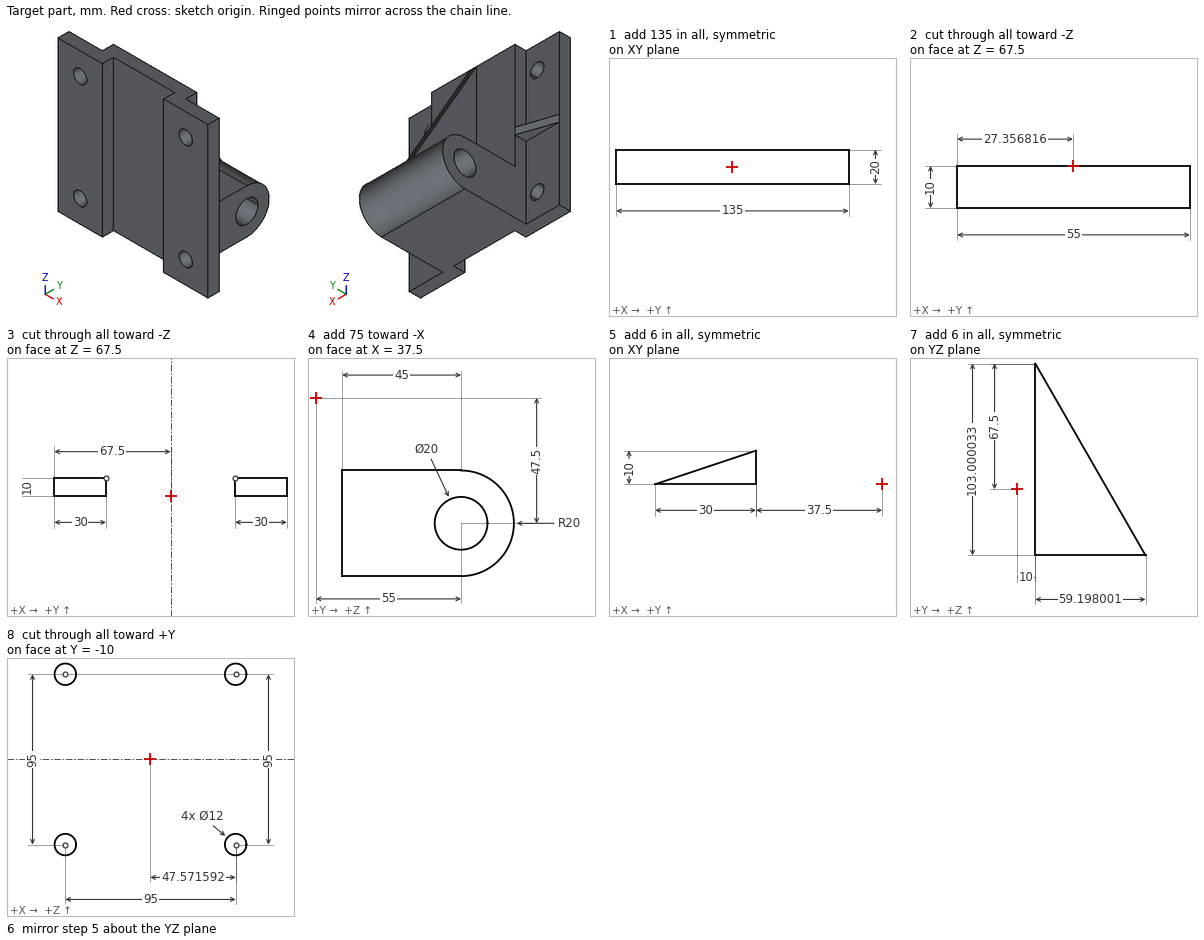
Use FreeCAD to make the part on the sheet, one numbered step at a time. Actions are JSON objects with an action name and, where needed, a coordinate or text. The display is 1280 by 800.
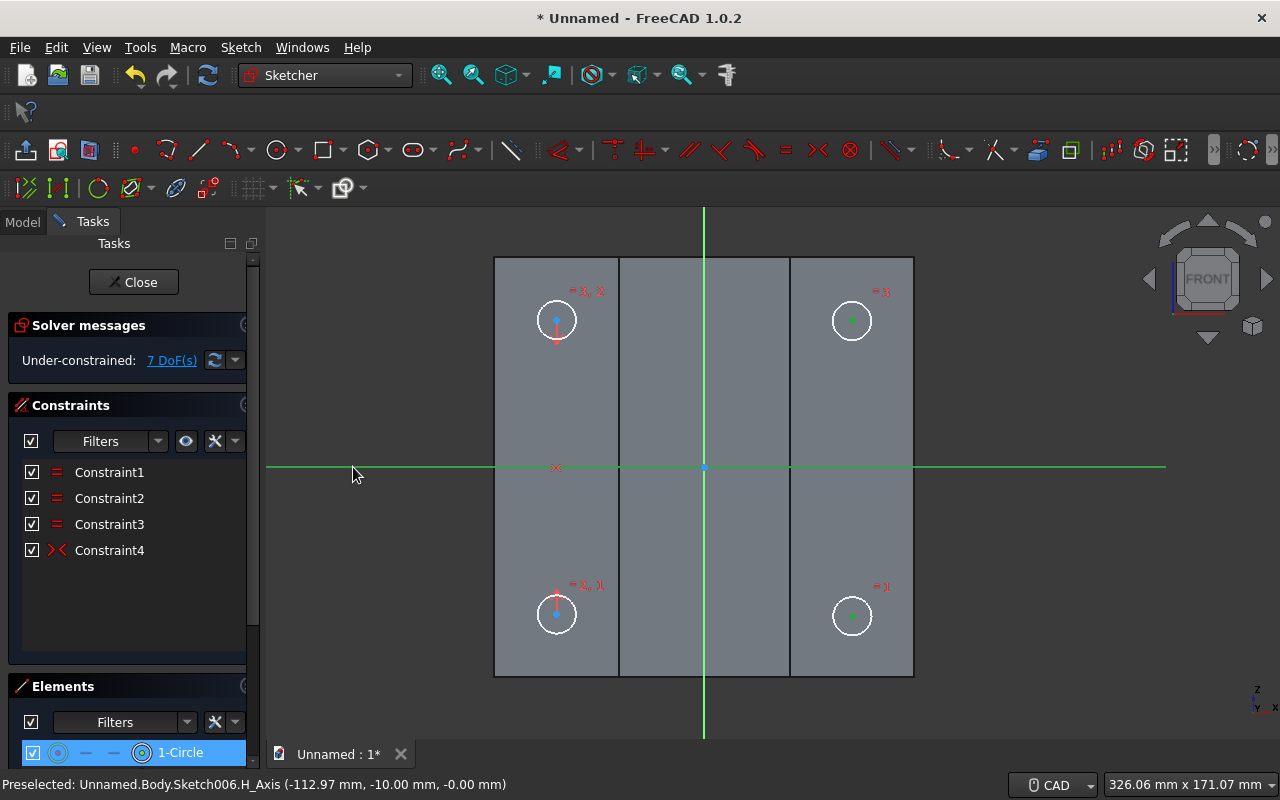
{"action": "left_click", "coordinate": [818, 150]}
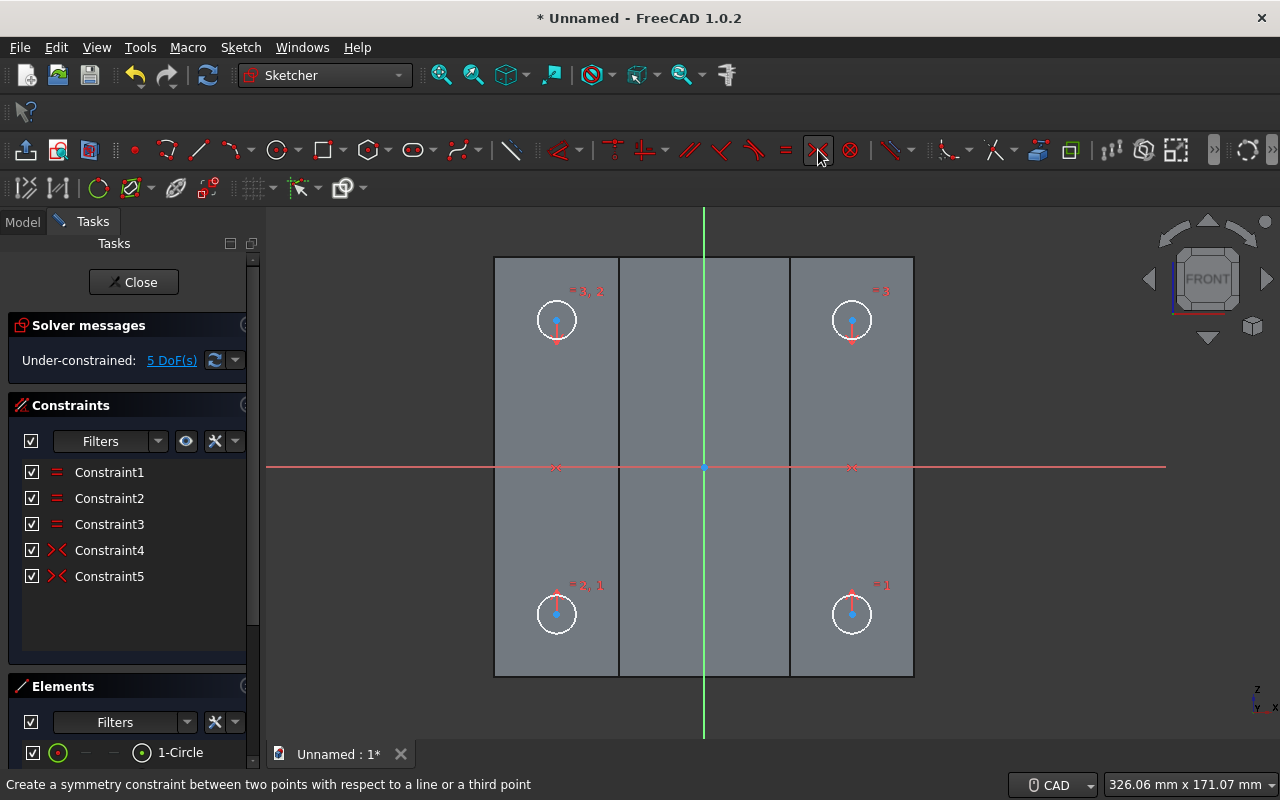
{"action": "left_click", "coordinate": [558, 150]}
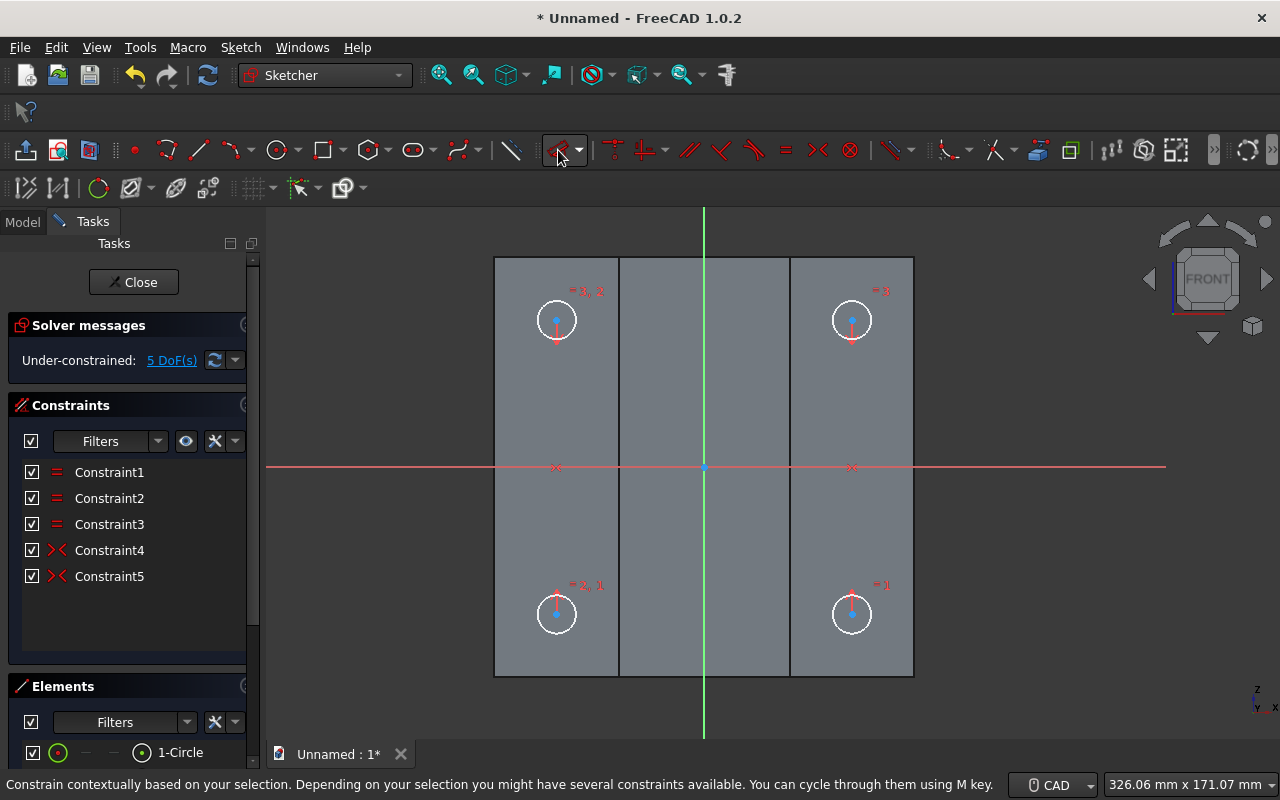
{"action": "left_click", "coordinate": [865, 601]}
{"action": "left_click", "coordinate": [887, 578]}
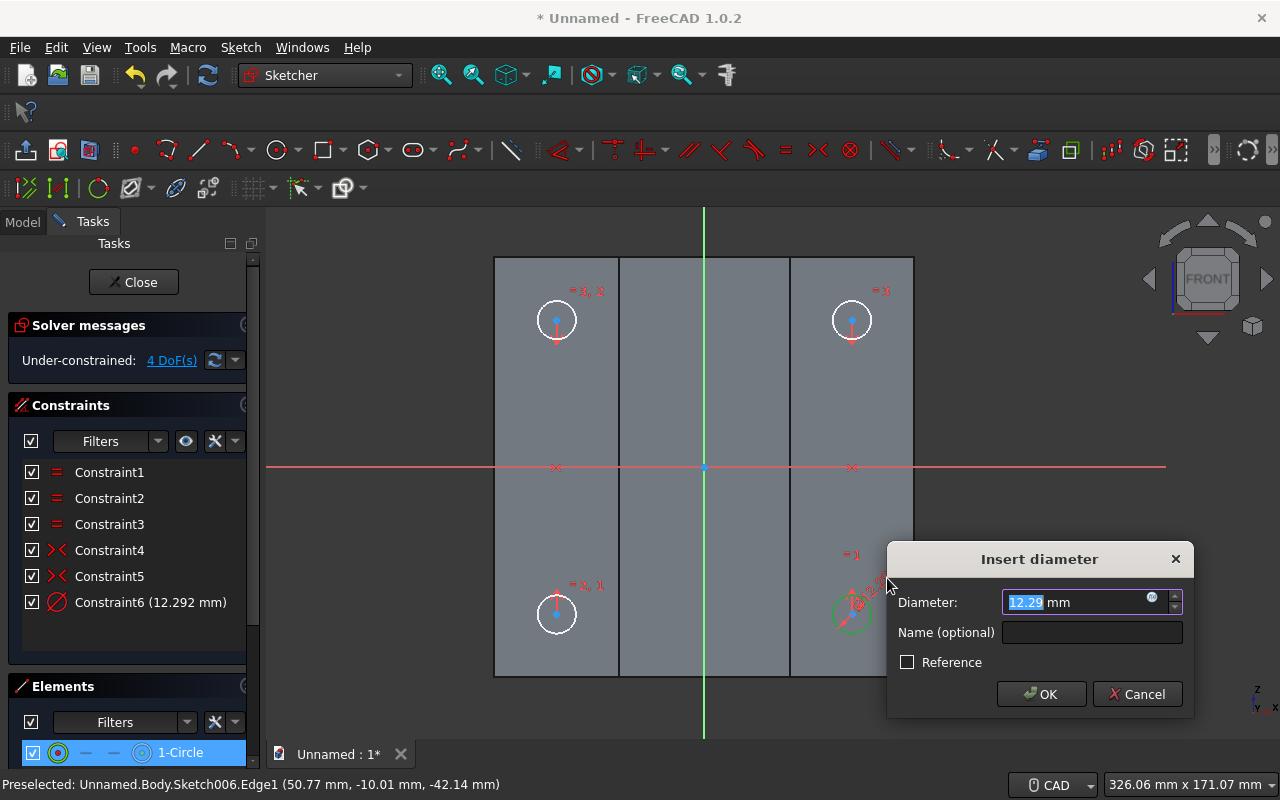
{"action": "type", "text": "12"}
{"action": "key", "text": "Return"}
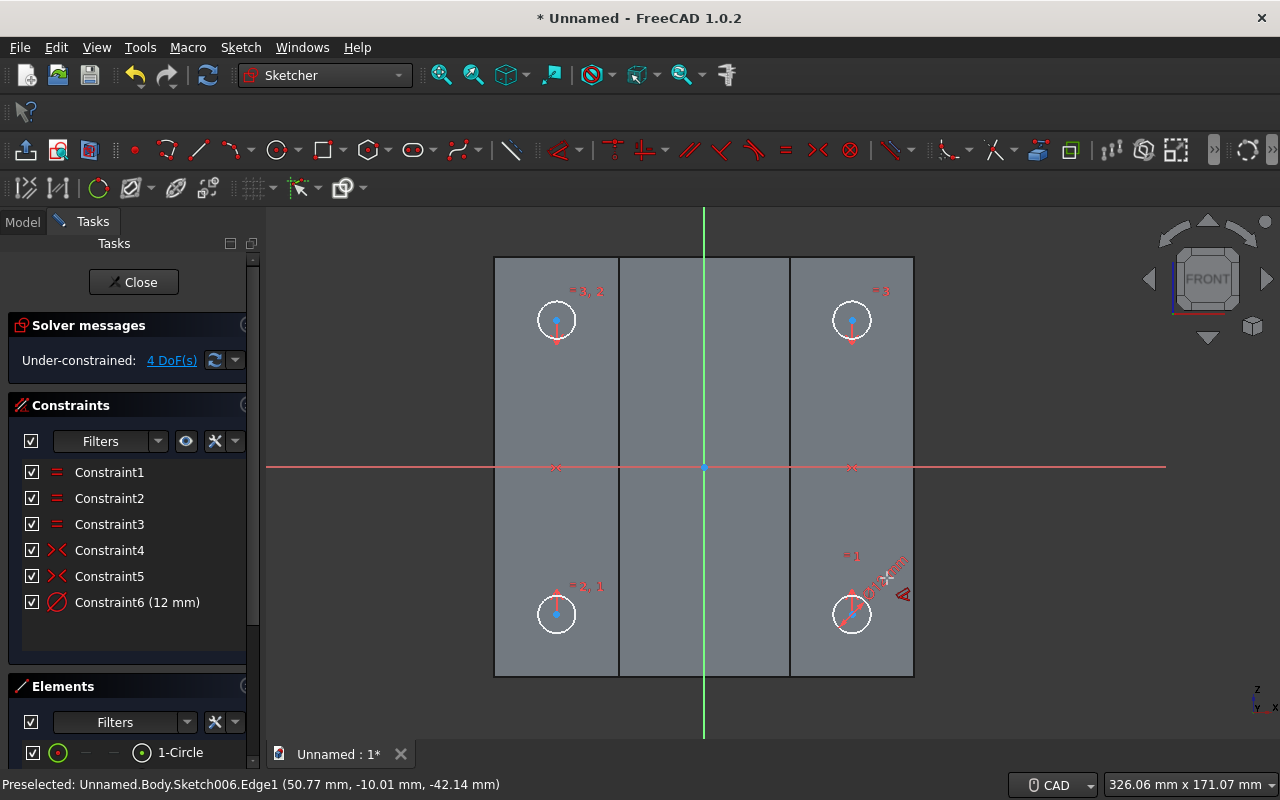
{"action": "left_click", "coordinate": [852, 614]}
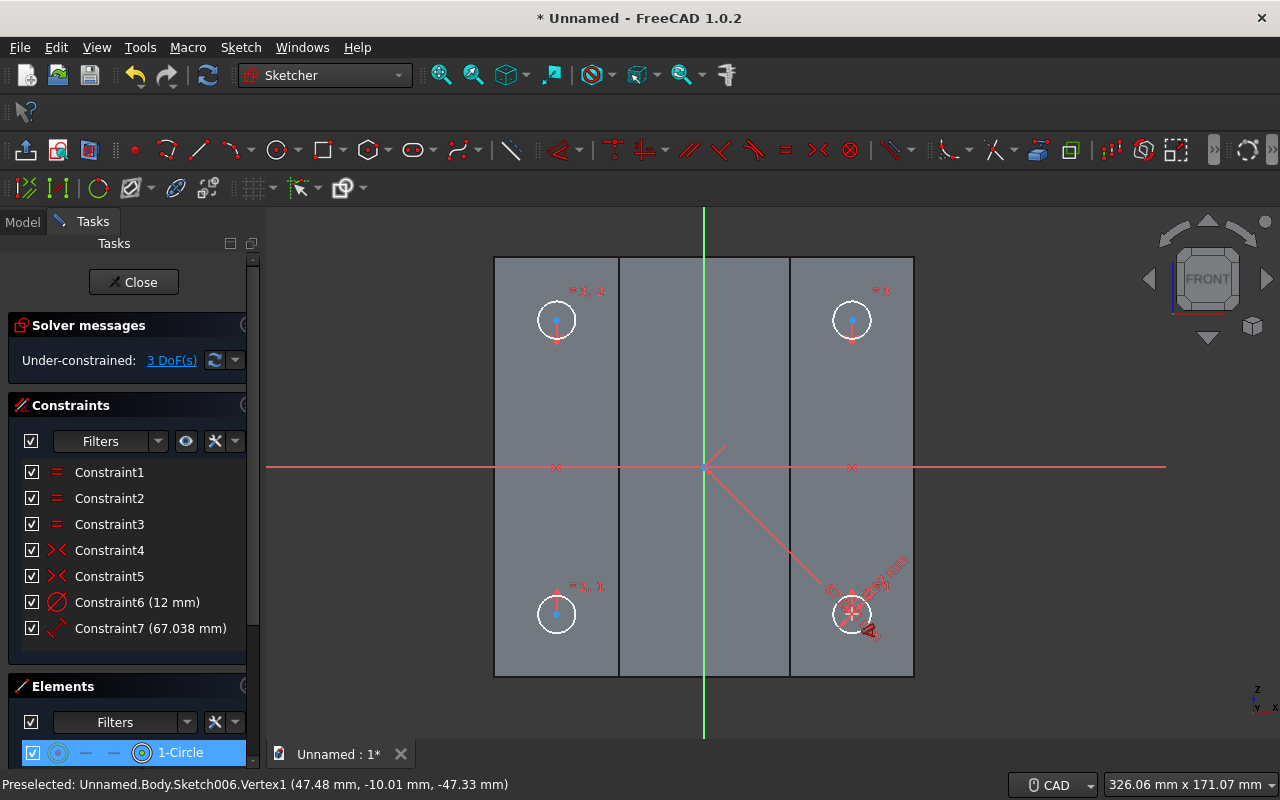
{"action": "left_click", "coordinate": [557, 614]}
{"action": "left_click", "coordinate": [637, 648]}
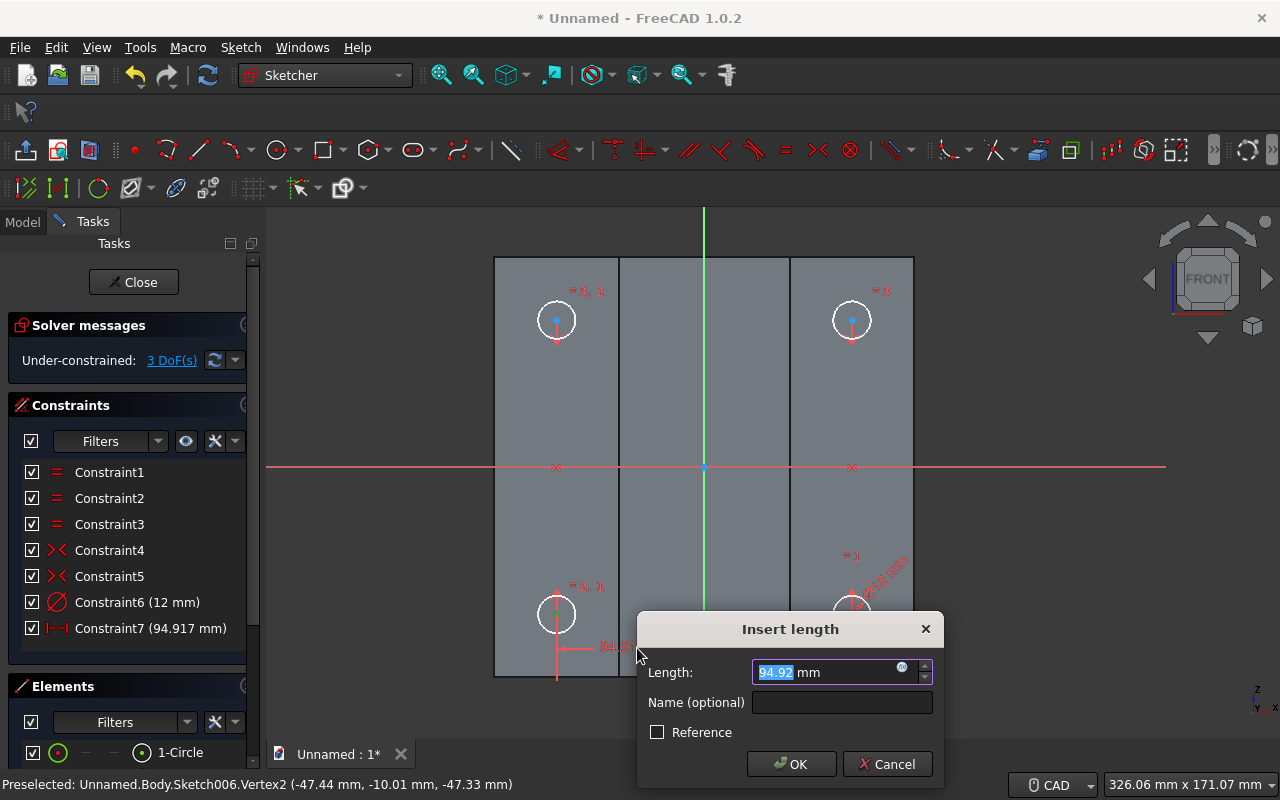
{"action": "type", "text": "95"}
{"action": "key", "text": "Return"}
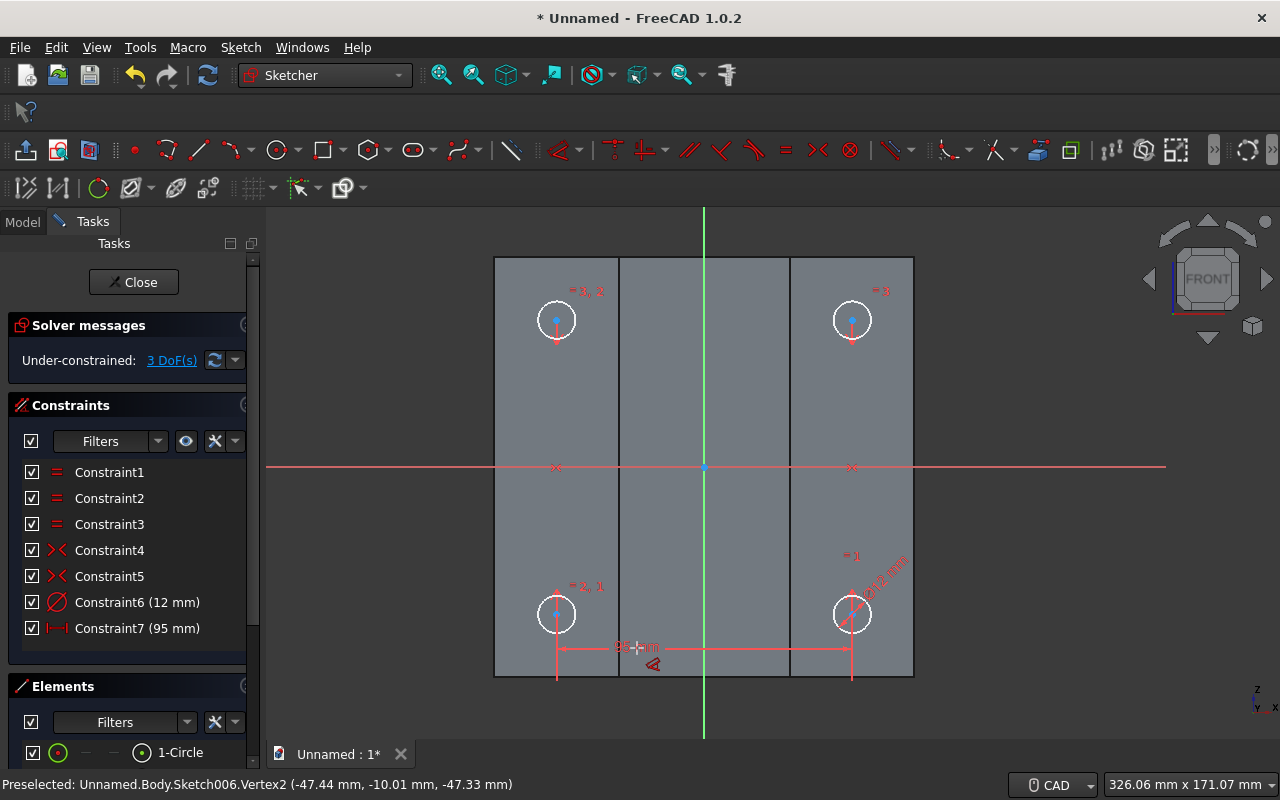
{"action": "left_click", "coordinate": [557, 614]}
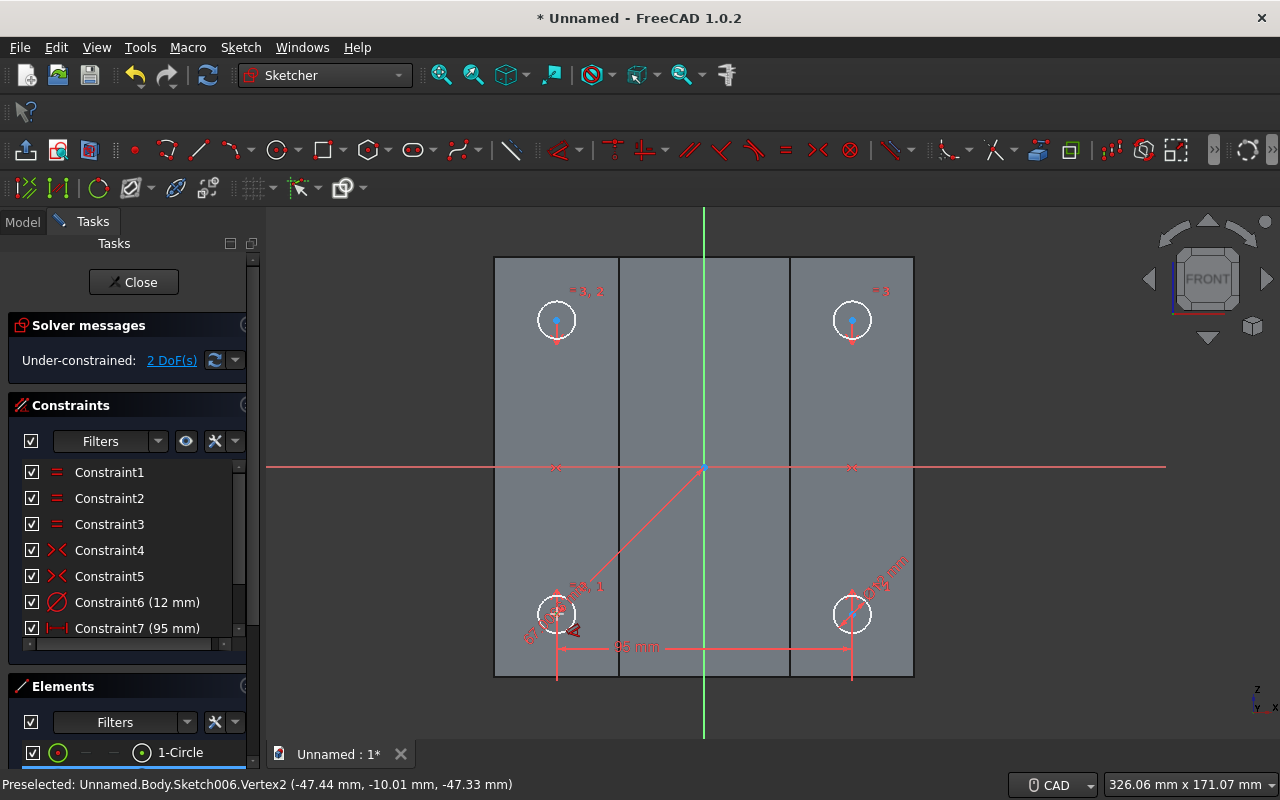
{"action": "left_click", "coordinate": [557, 320]}
{"action": "left_click", "coordinate": [523, 400]}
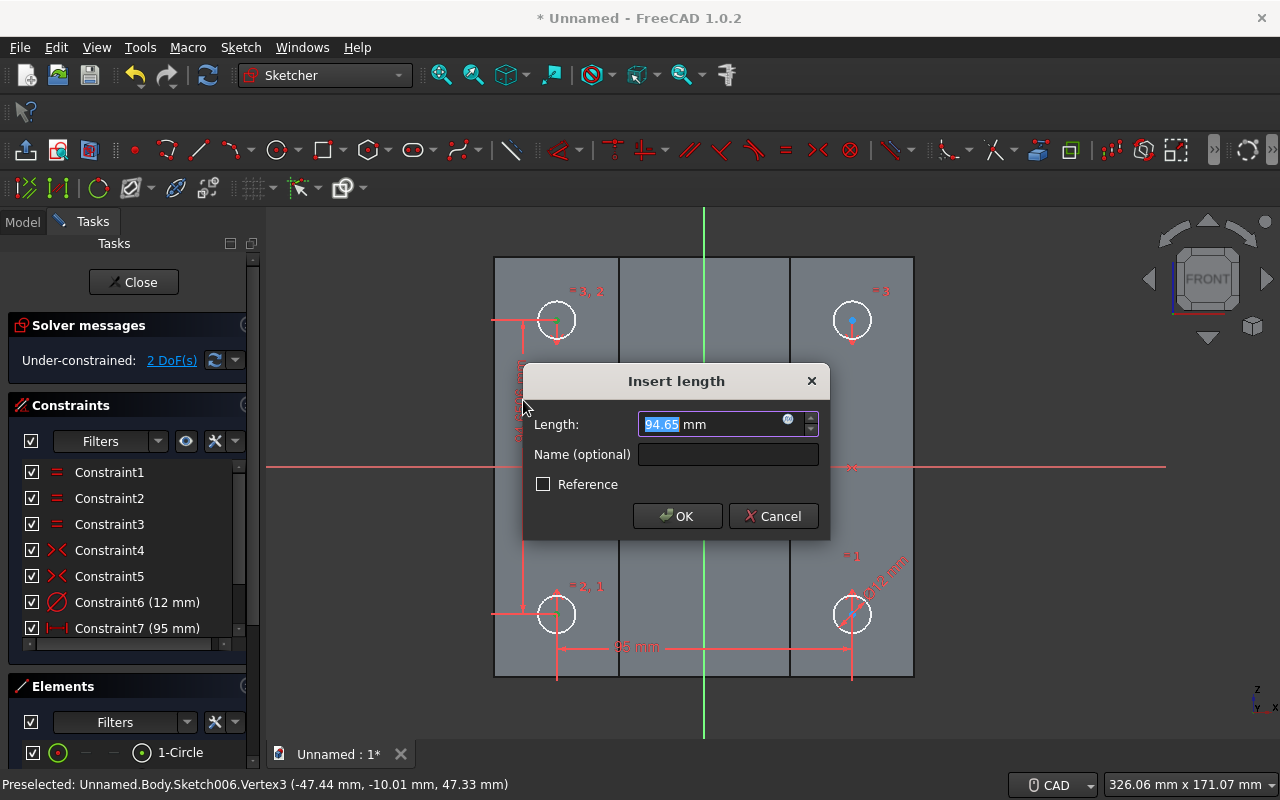
{"action": "type", "text": "95"}
{"action": "key", "text": "Return"}